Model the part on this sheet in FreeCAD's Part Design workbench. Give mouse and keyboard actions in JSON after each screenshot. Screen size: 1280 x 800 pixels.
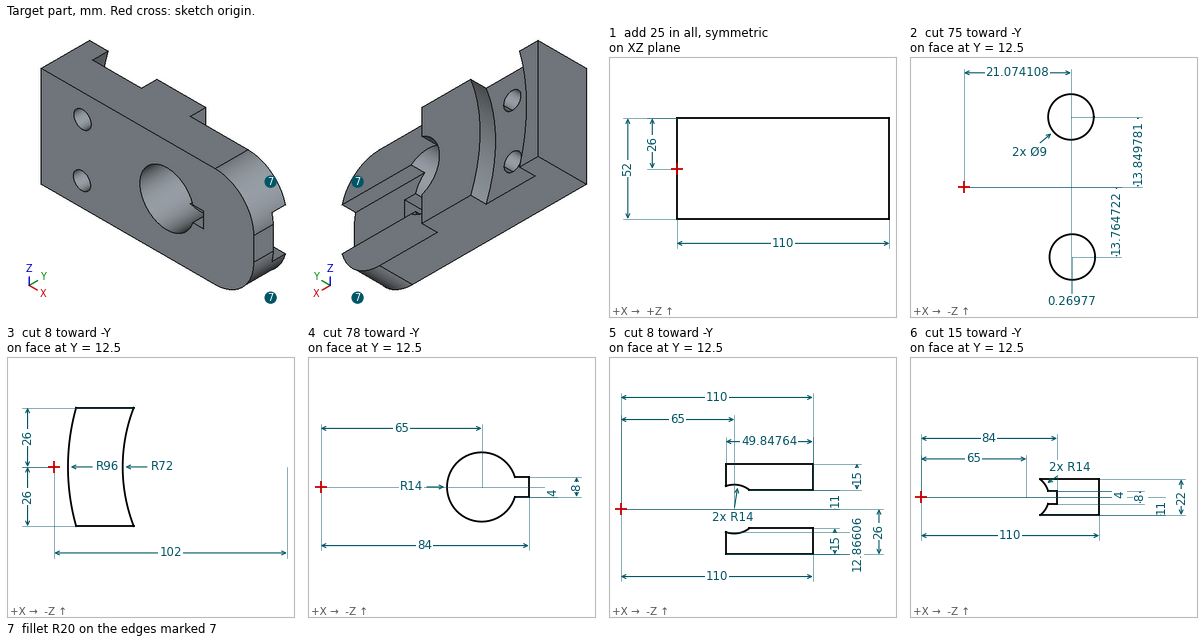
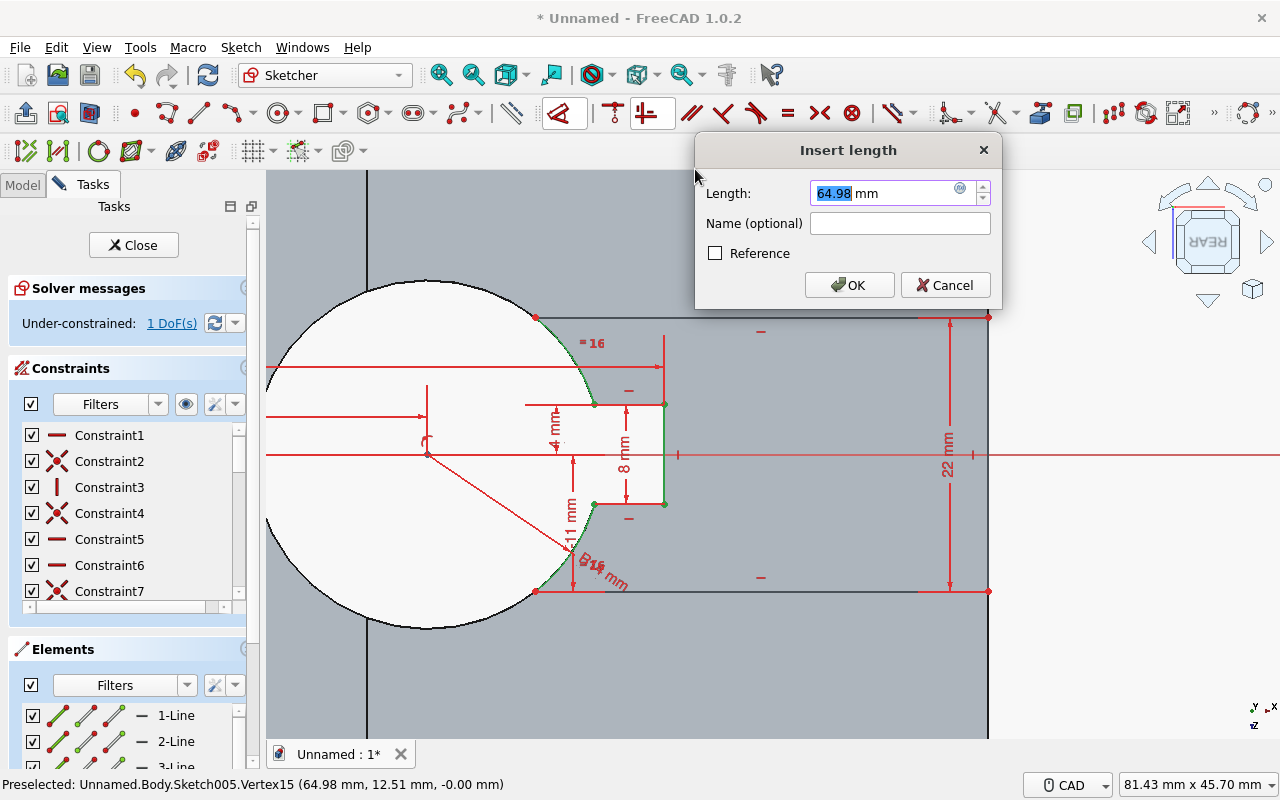
{"action": "type", "text": "65"}
{"action": "key", "text": "Return"}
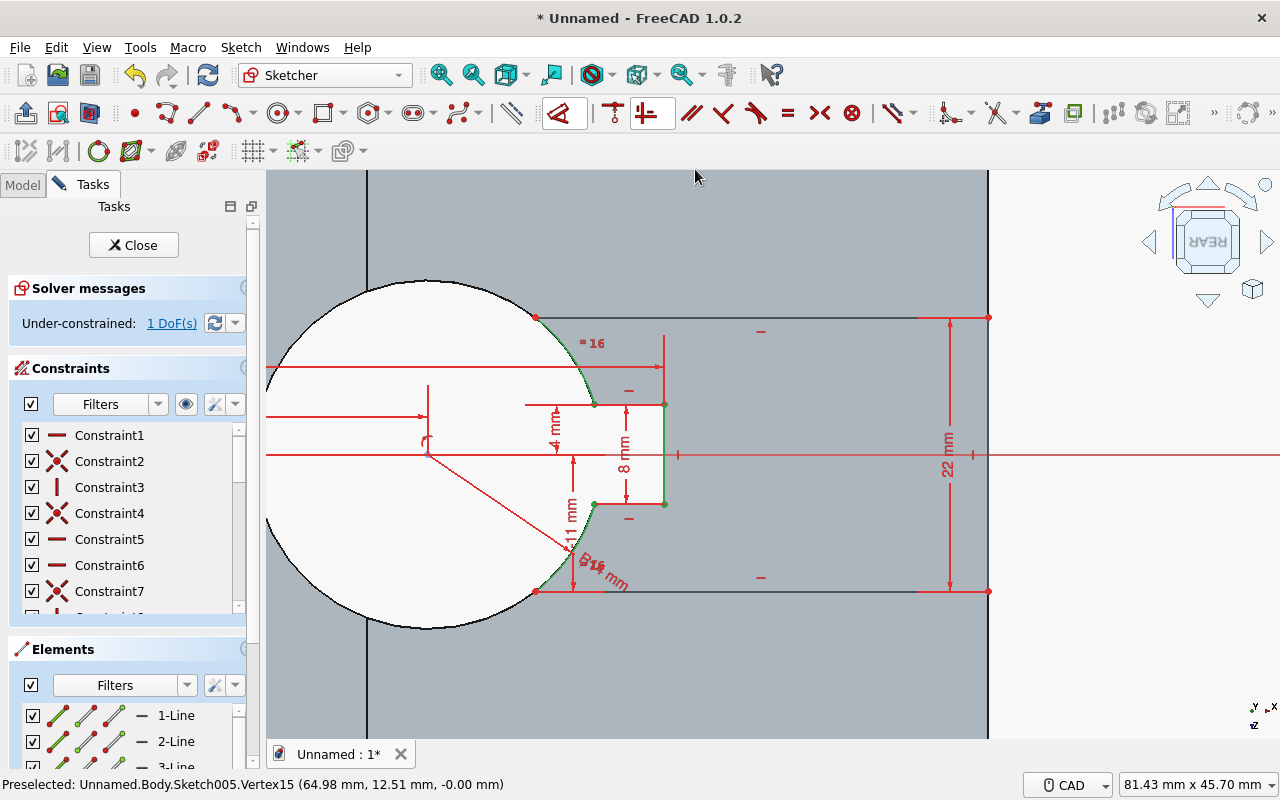
{"action": "left_click", "coordinate": [988, 592]}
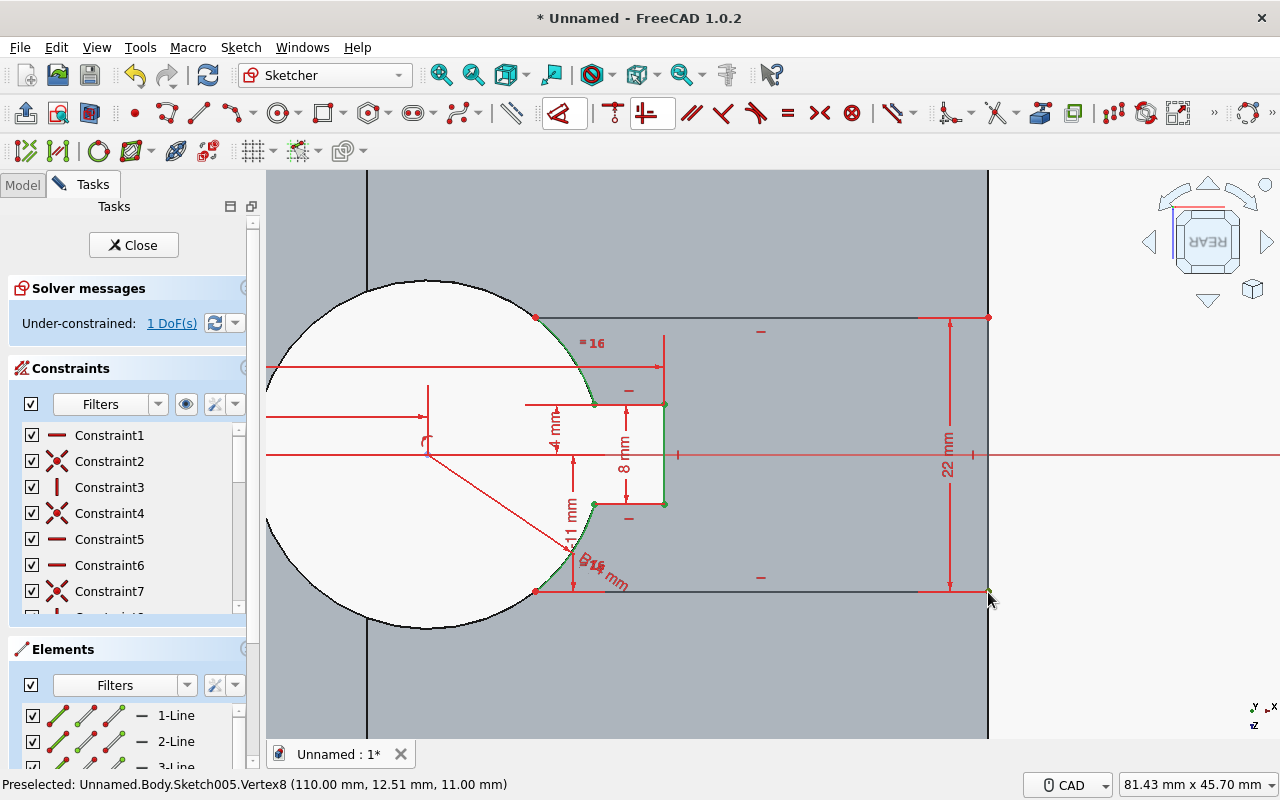
{"action": "left_click", "coordinate": [582, 114]}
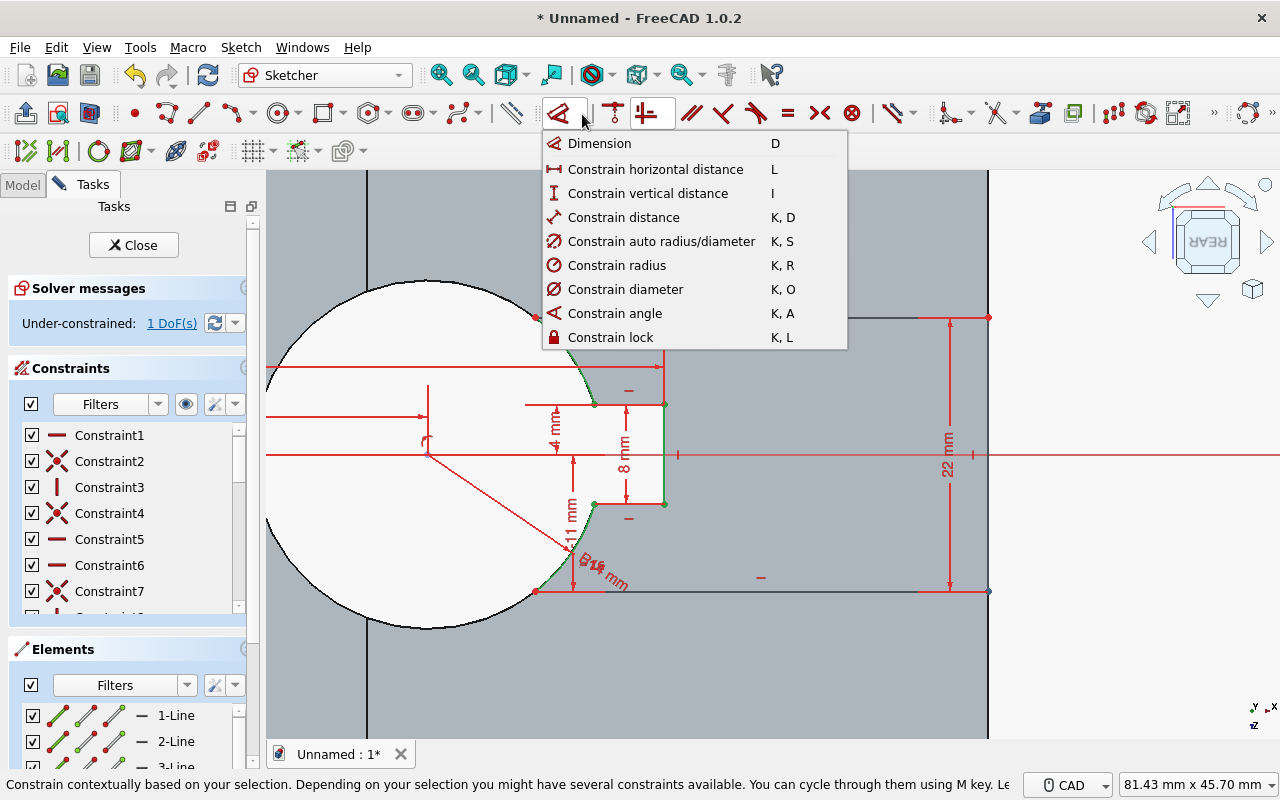
{"action": "left_click", "coordinate": [695, 169]}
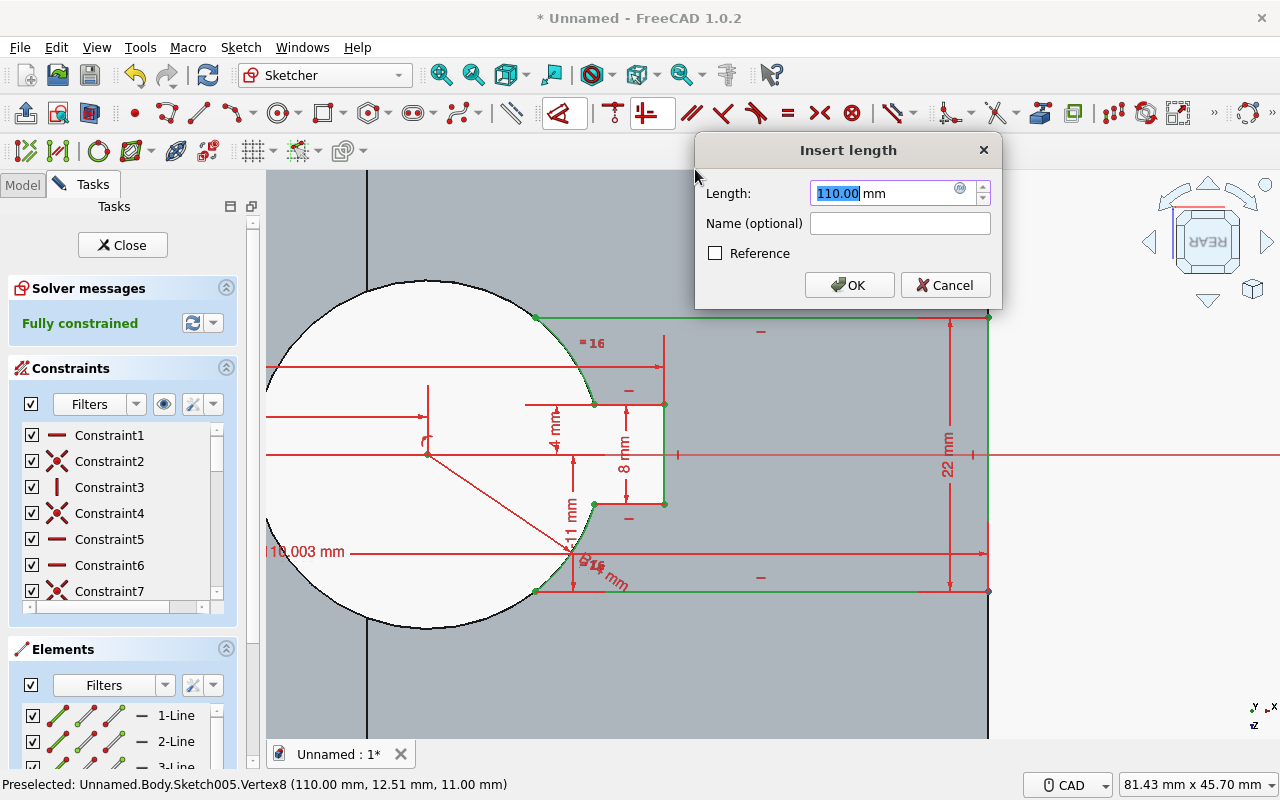
{"action": "type", "text": "110"}
{"action": "key", "text": "Return"}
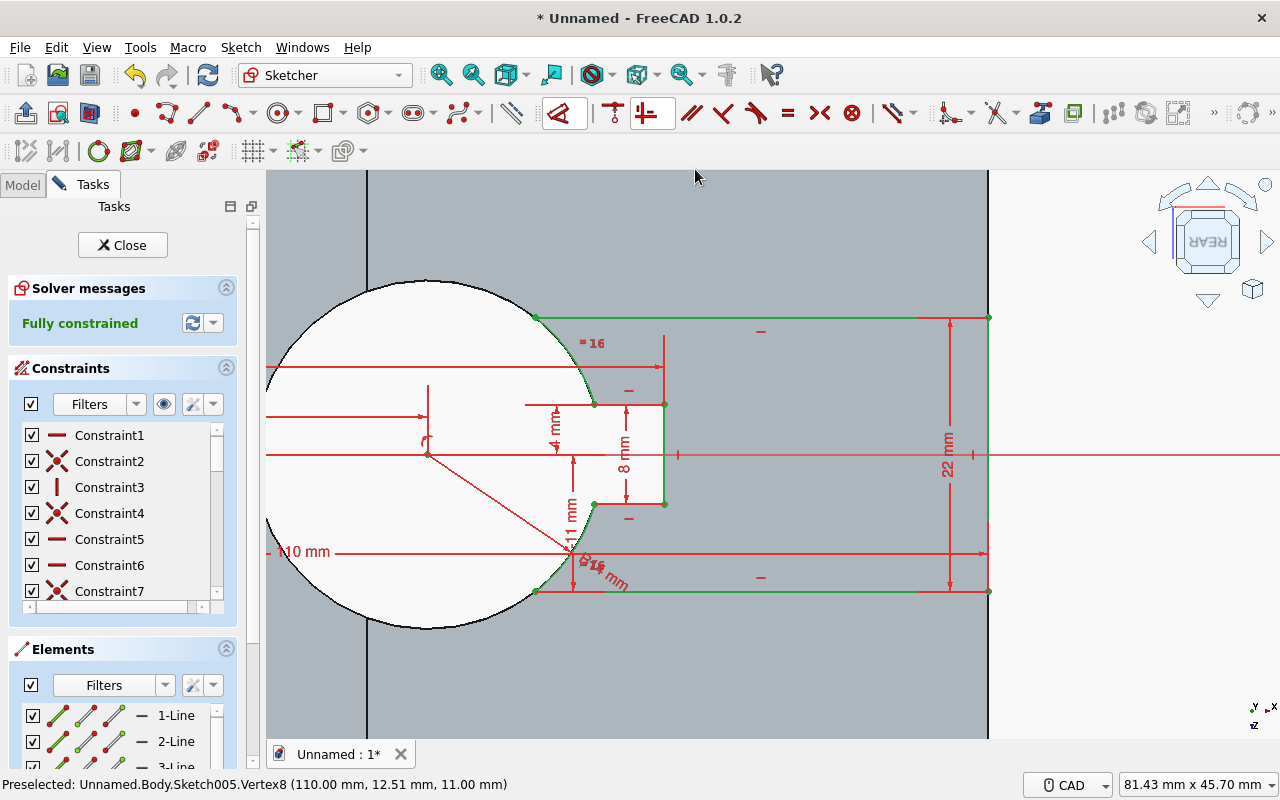
{"action": "left_click", "coordinate": [123, 245]}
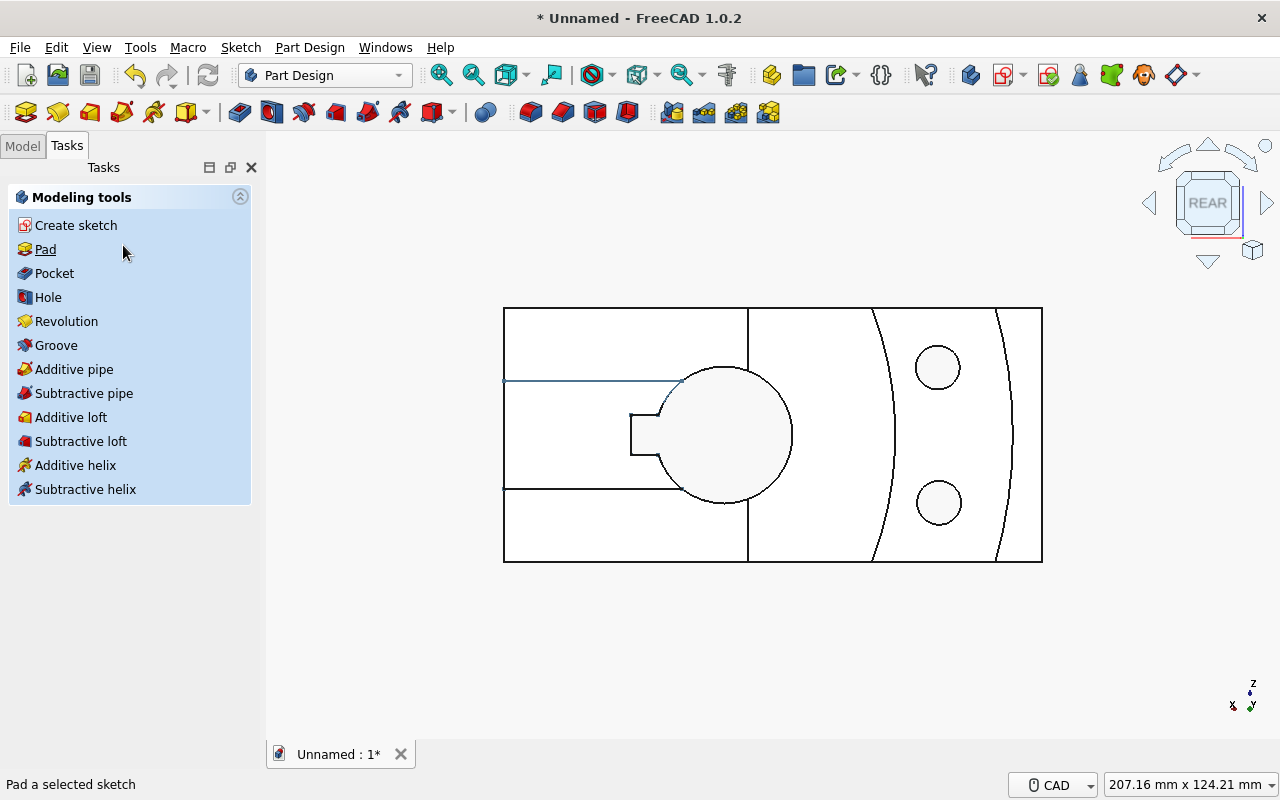
{"action": "left_click", "coordinate": [240, 112]}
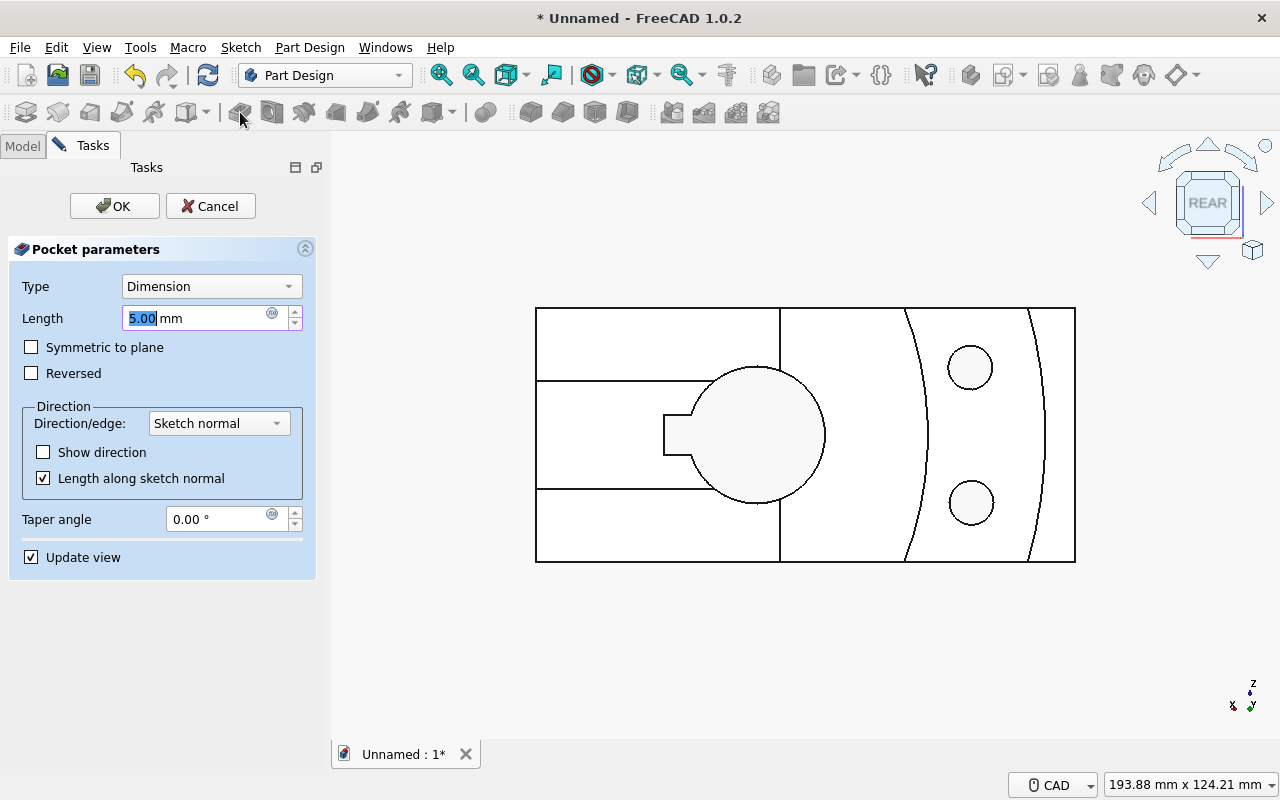
{"action": "type", "text": "15"}
{"action": "key", "text": "Tab"}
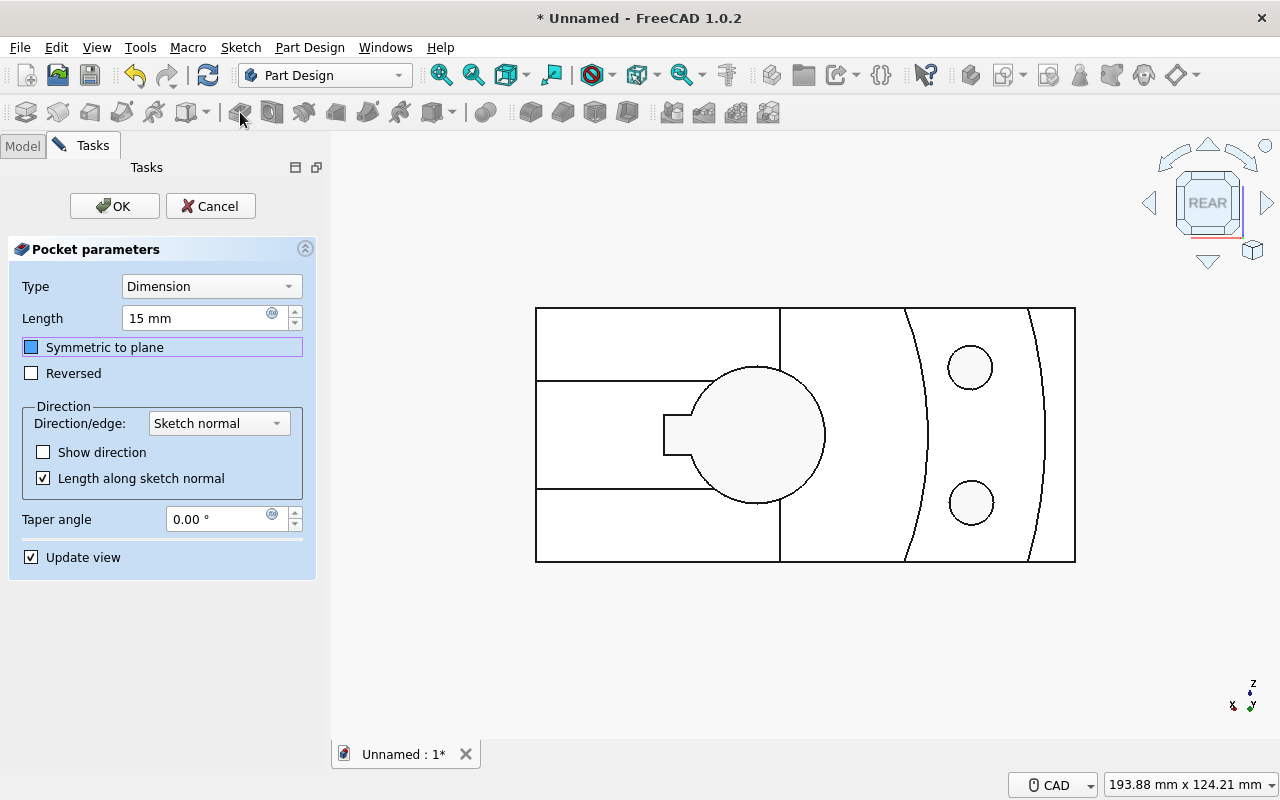
{"action": "left_click", "coordinate": [115, 206]}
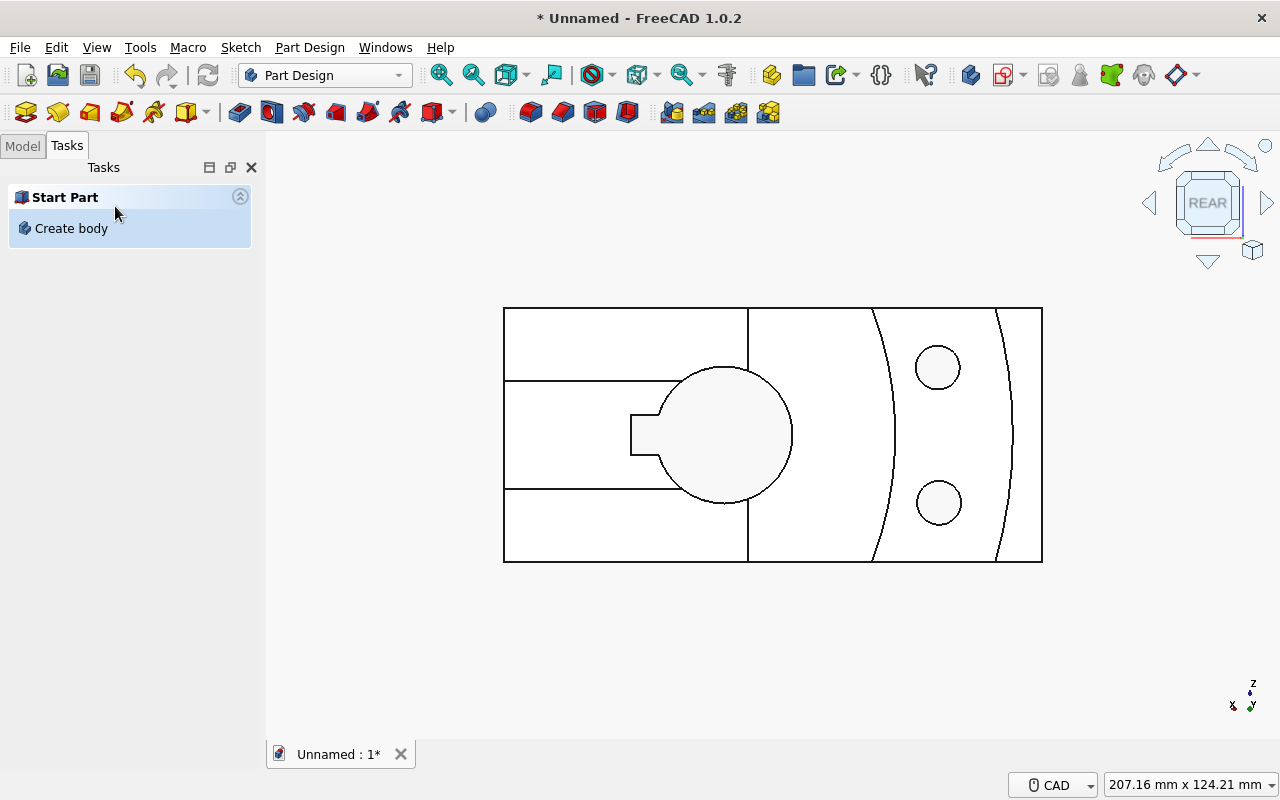
{"action": "key", "text": "0"}